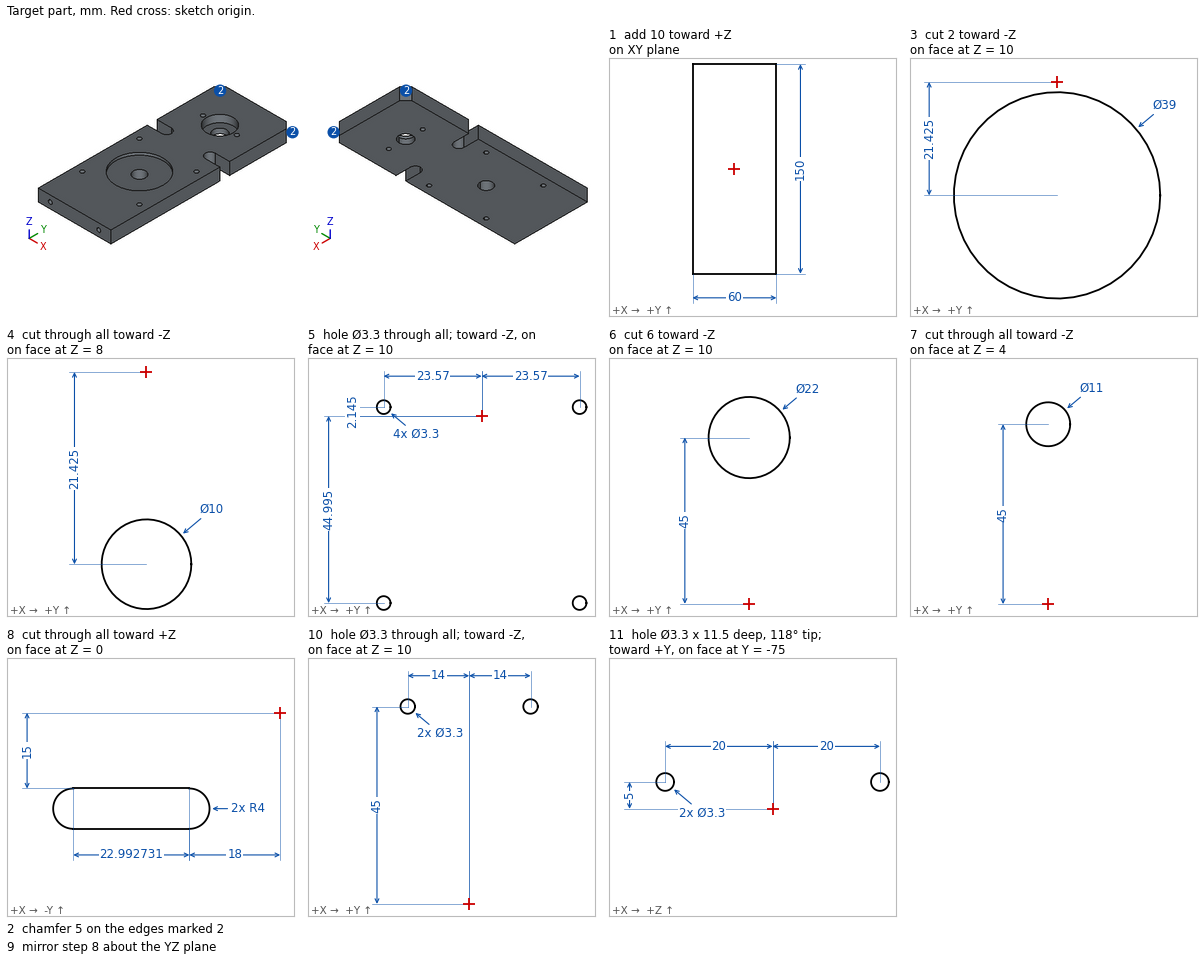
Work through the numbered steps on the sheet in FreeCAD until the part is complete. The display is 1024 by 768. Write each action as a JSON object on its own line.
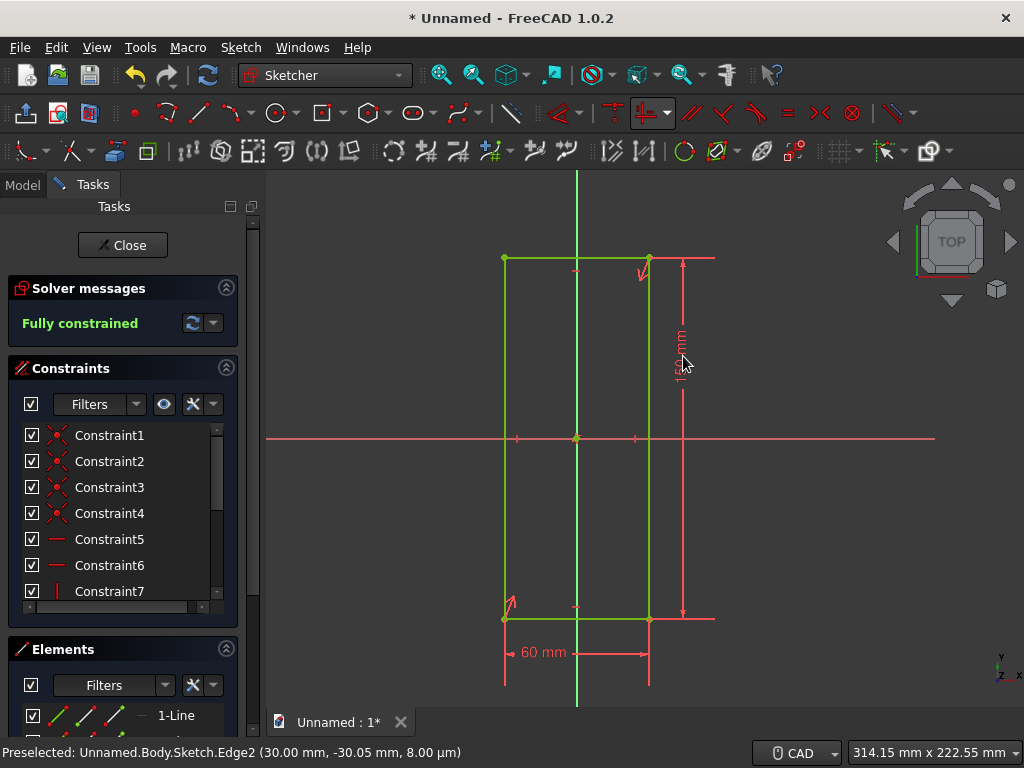
{"action": "left_click", "coordinate": [123, 245]}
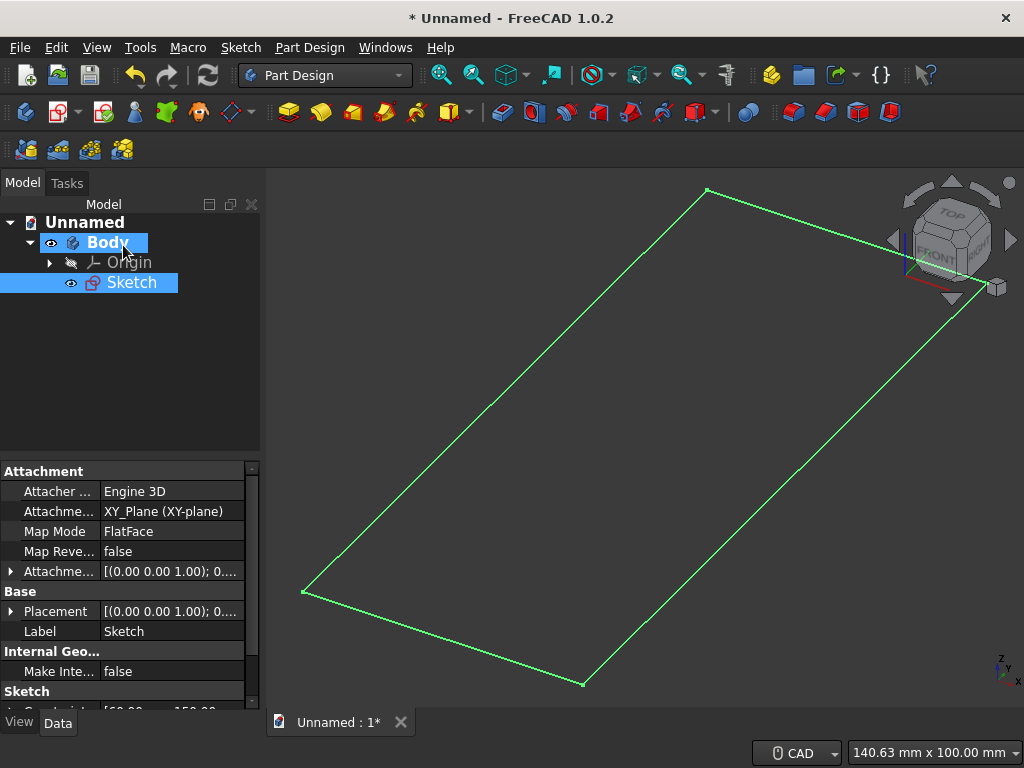
{"action": "left_click", "coordinate": [290, 112]}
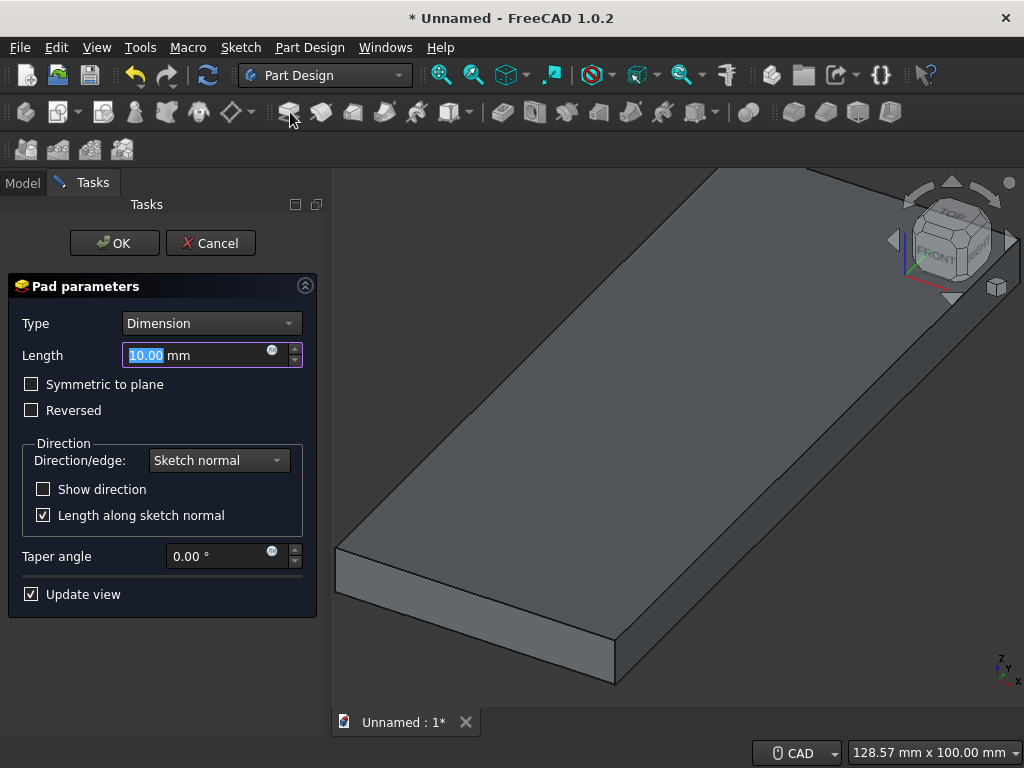
{"action": "type", "text": "10"}
{"action": "key", "text": "Tab"}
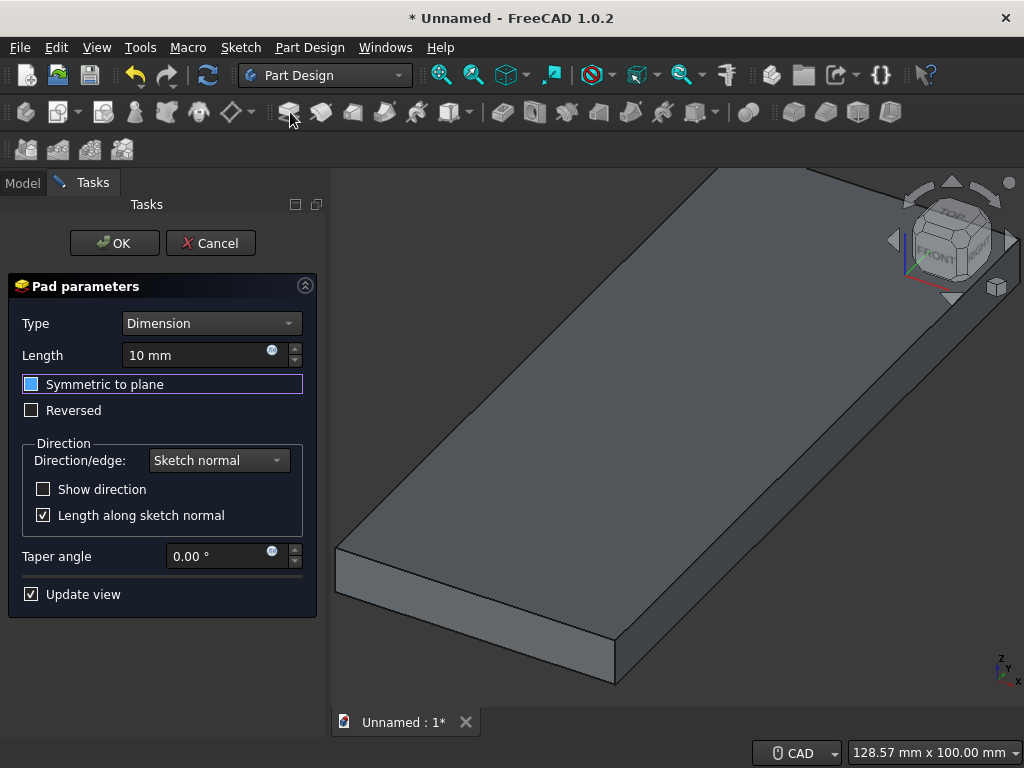
{"action": "left_click", "coordinate": [115, 243]}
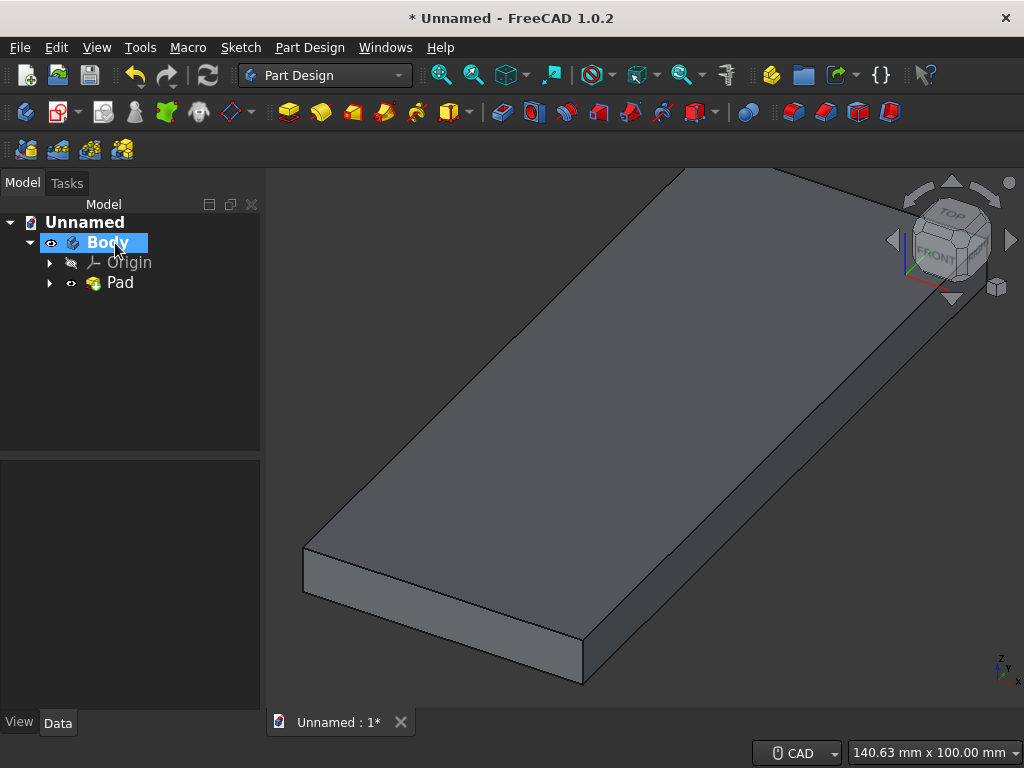
{"action": "left_click", "coordinate": [442, 76]}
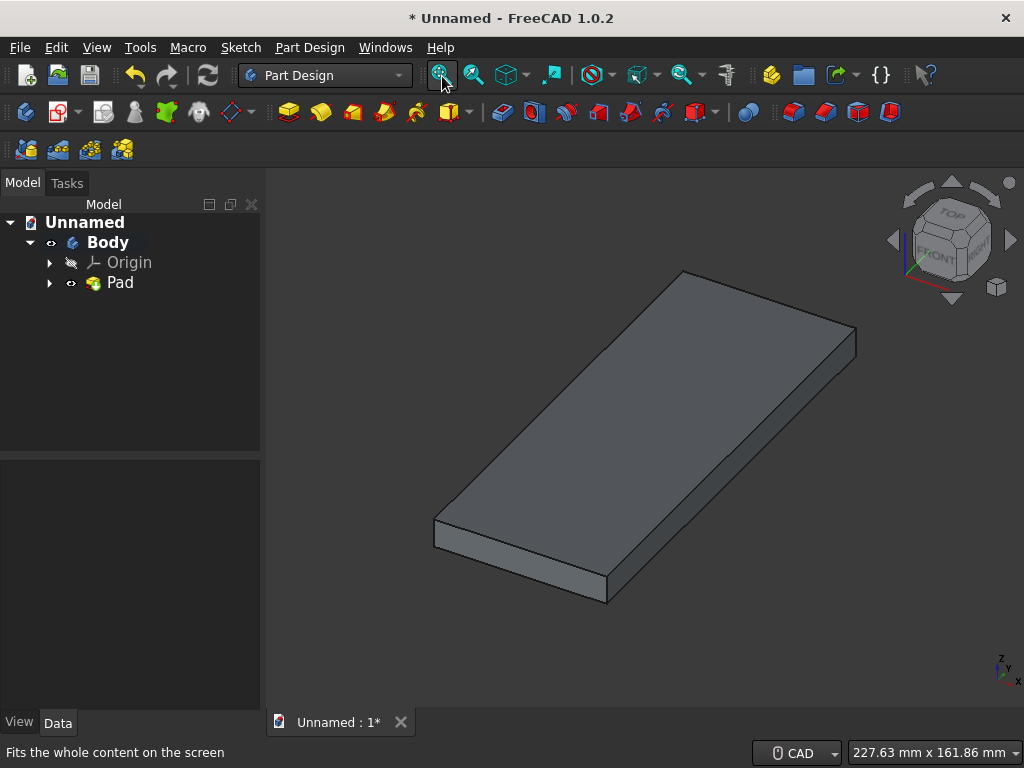
{"action": "key", "text": "0"}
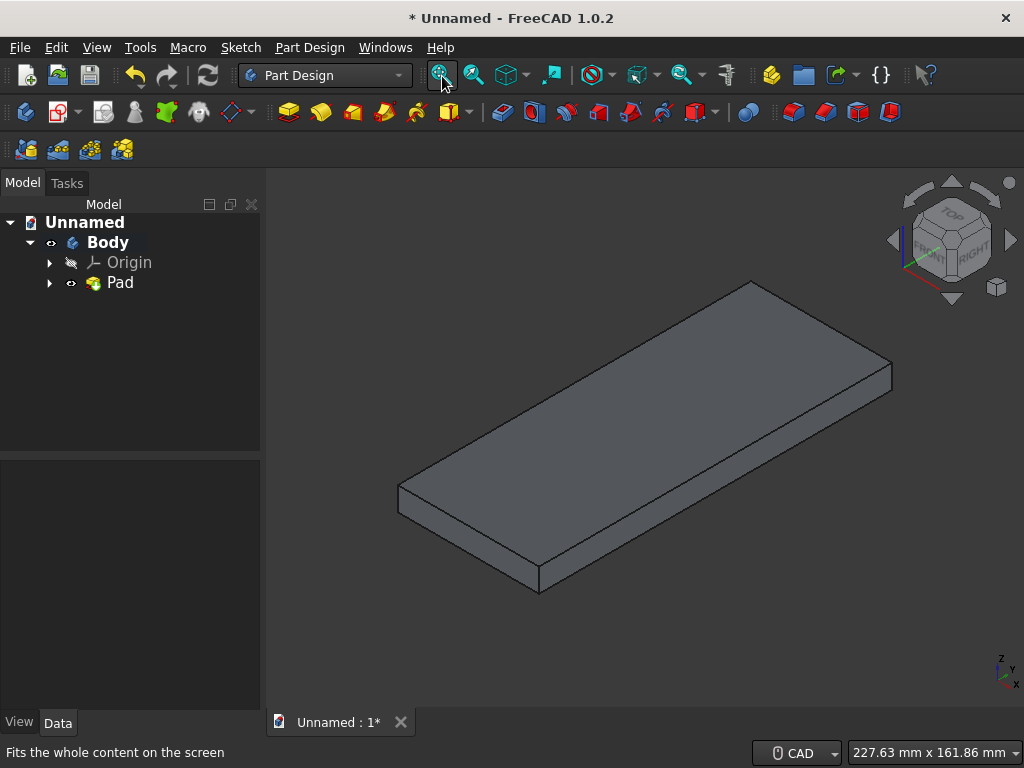
{"action": "key", "text": "2"}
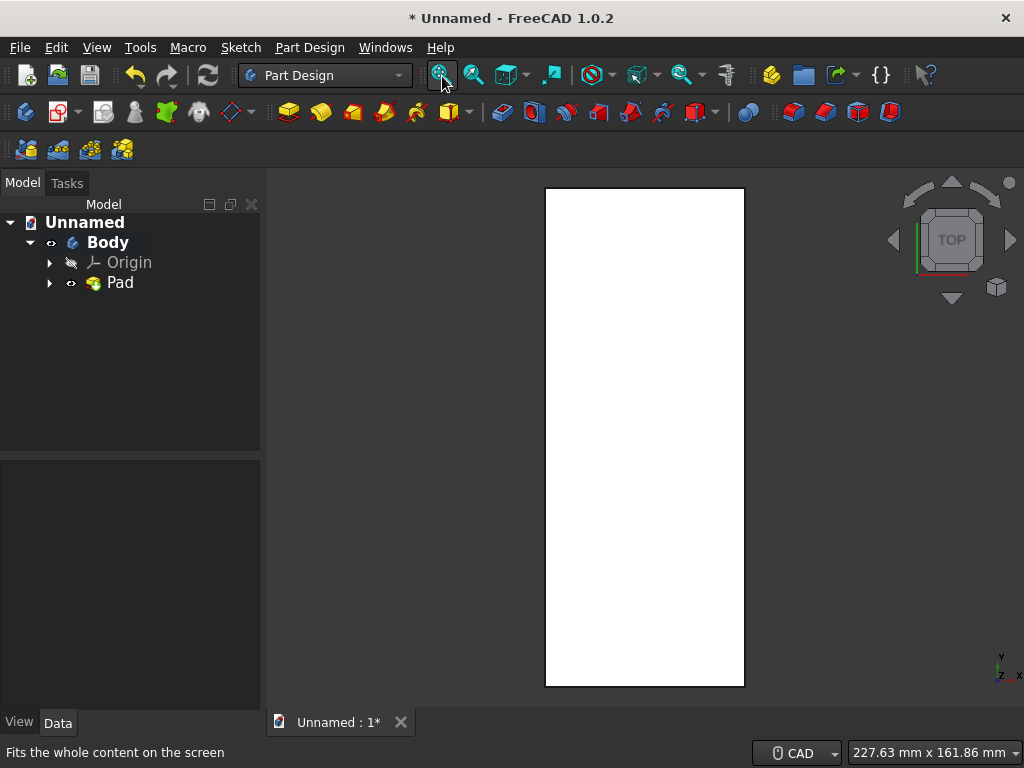
{"action": "key", "text": "1"}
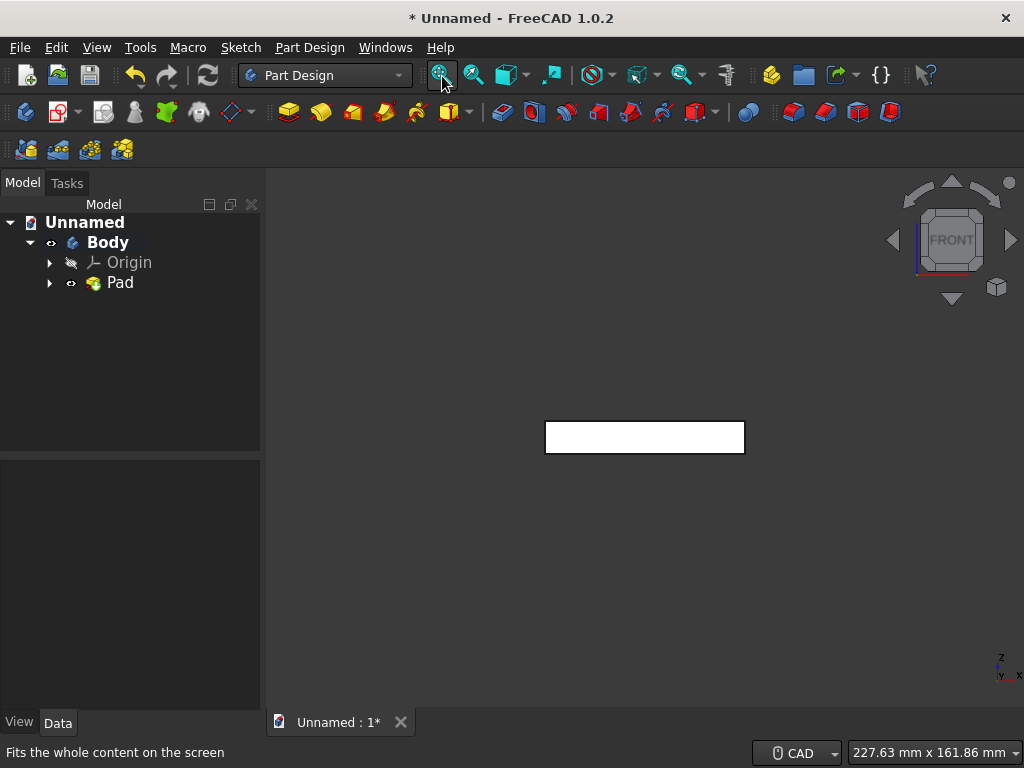
{"action": "left_click", "coordinate": [442, 76]}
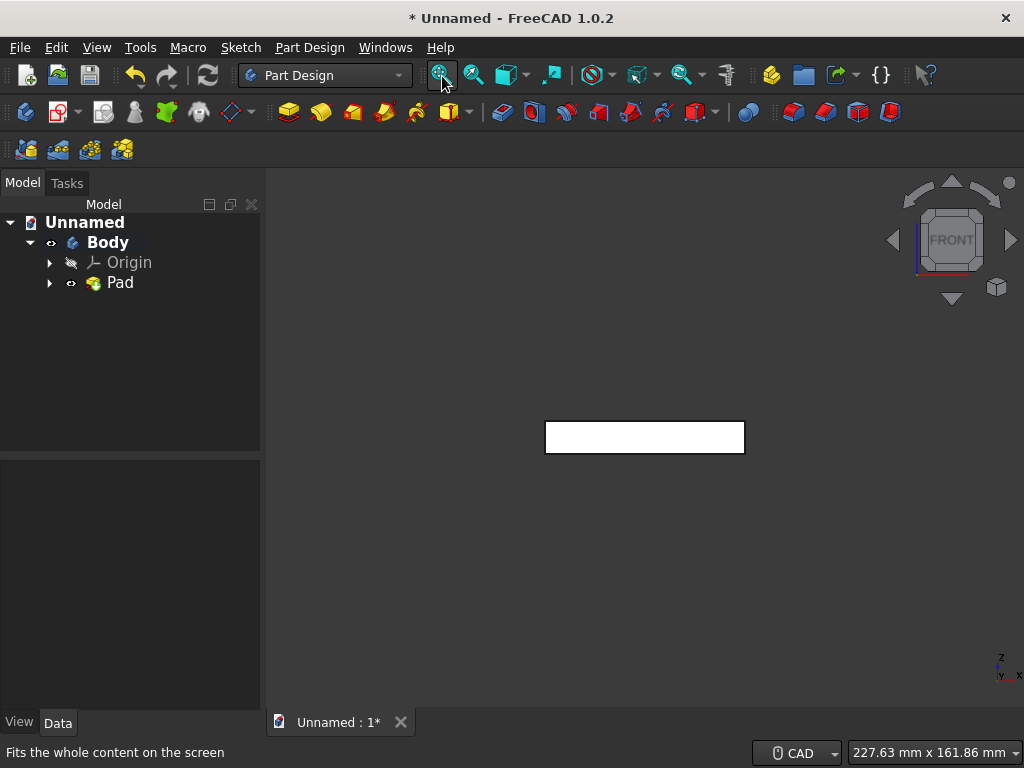
{"action": "key", "text": "3"}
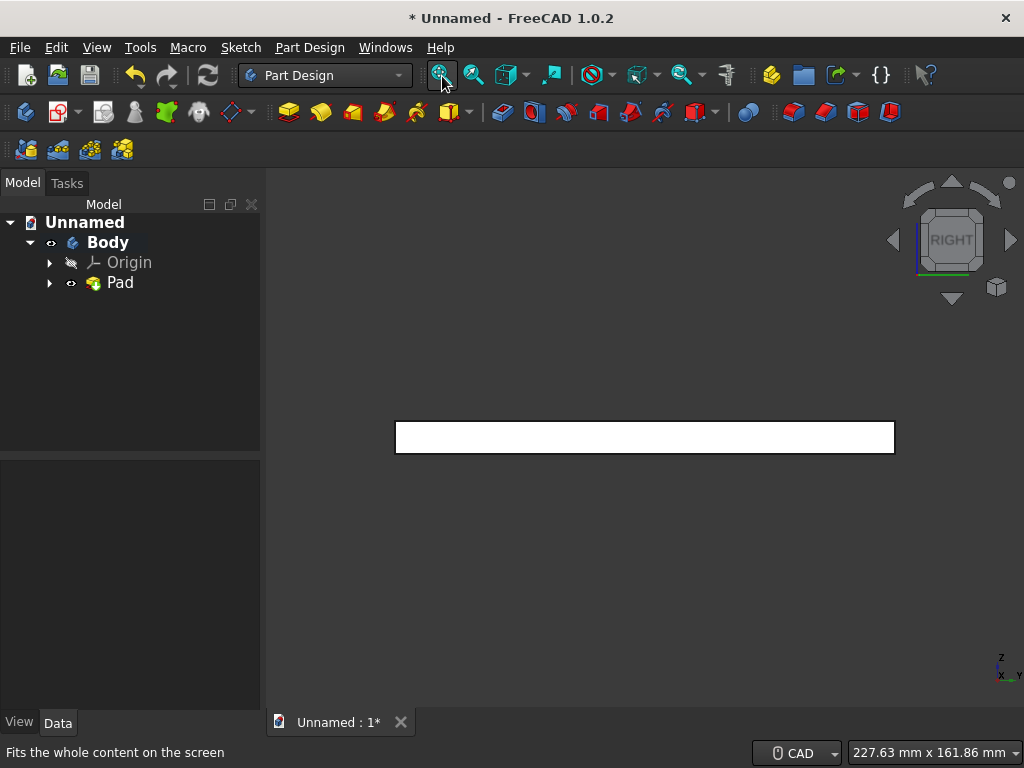
{"action": "left_click", "coordinate": [895, 436]}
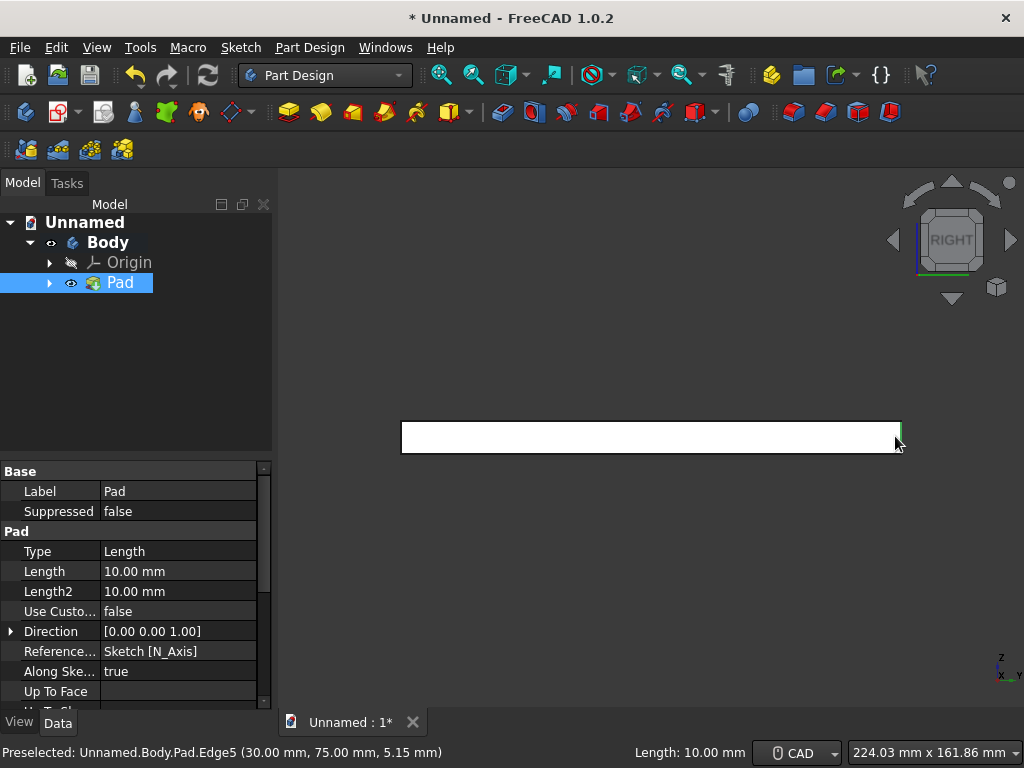
{"action": "key", "text": "5"}